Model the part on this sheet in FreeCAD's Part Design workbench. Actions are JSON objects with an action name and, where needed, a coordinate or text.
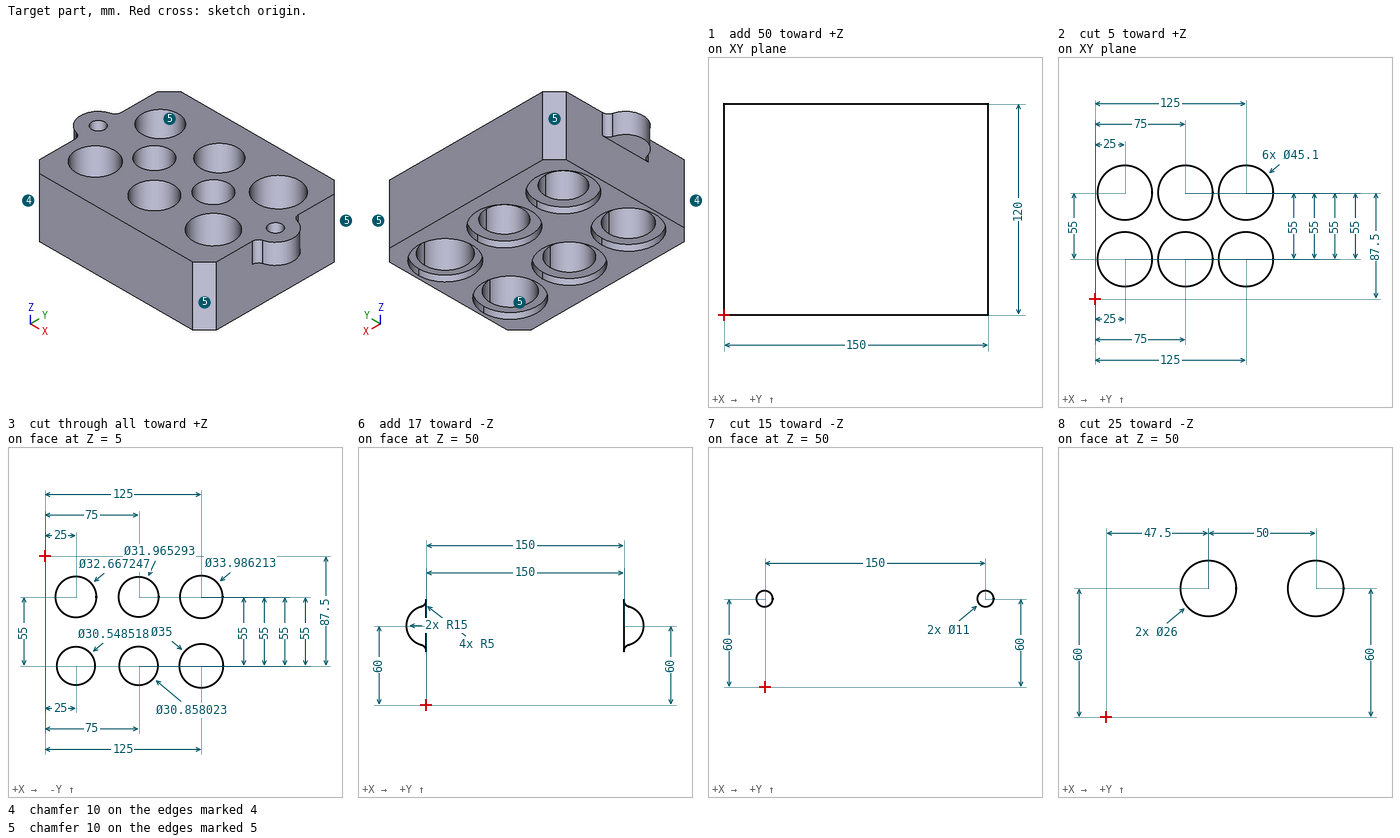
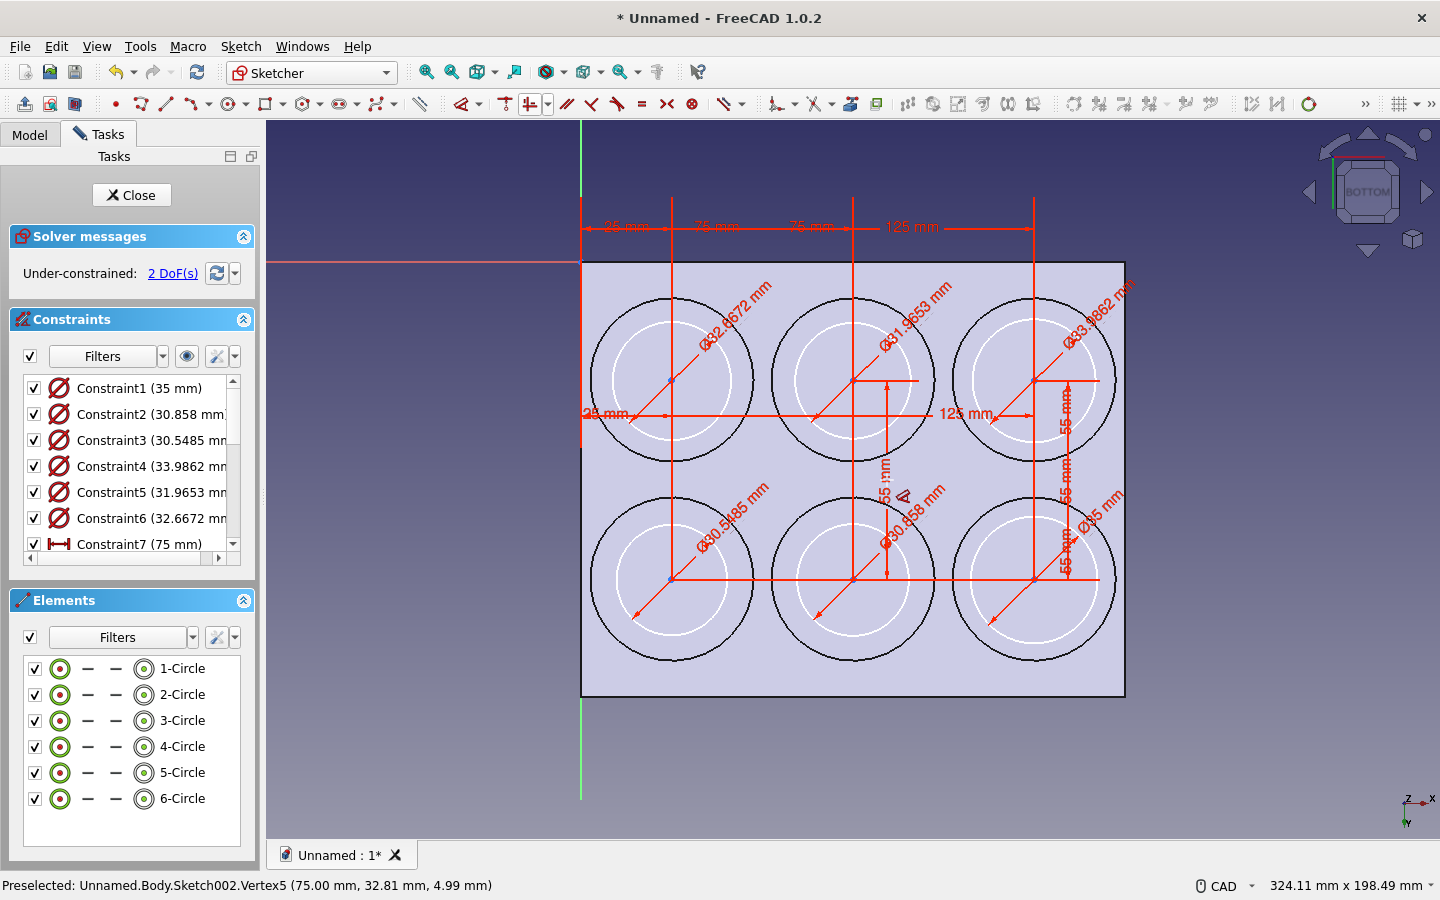
{"action": "left_click", "coordinate": [672, 580]}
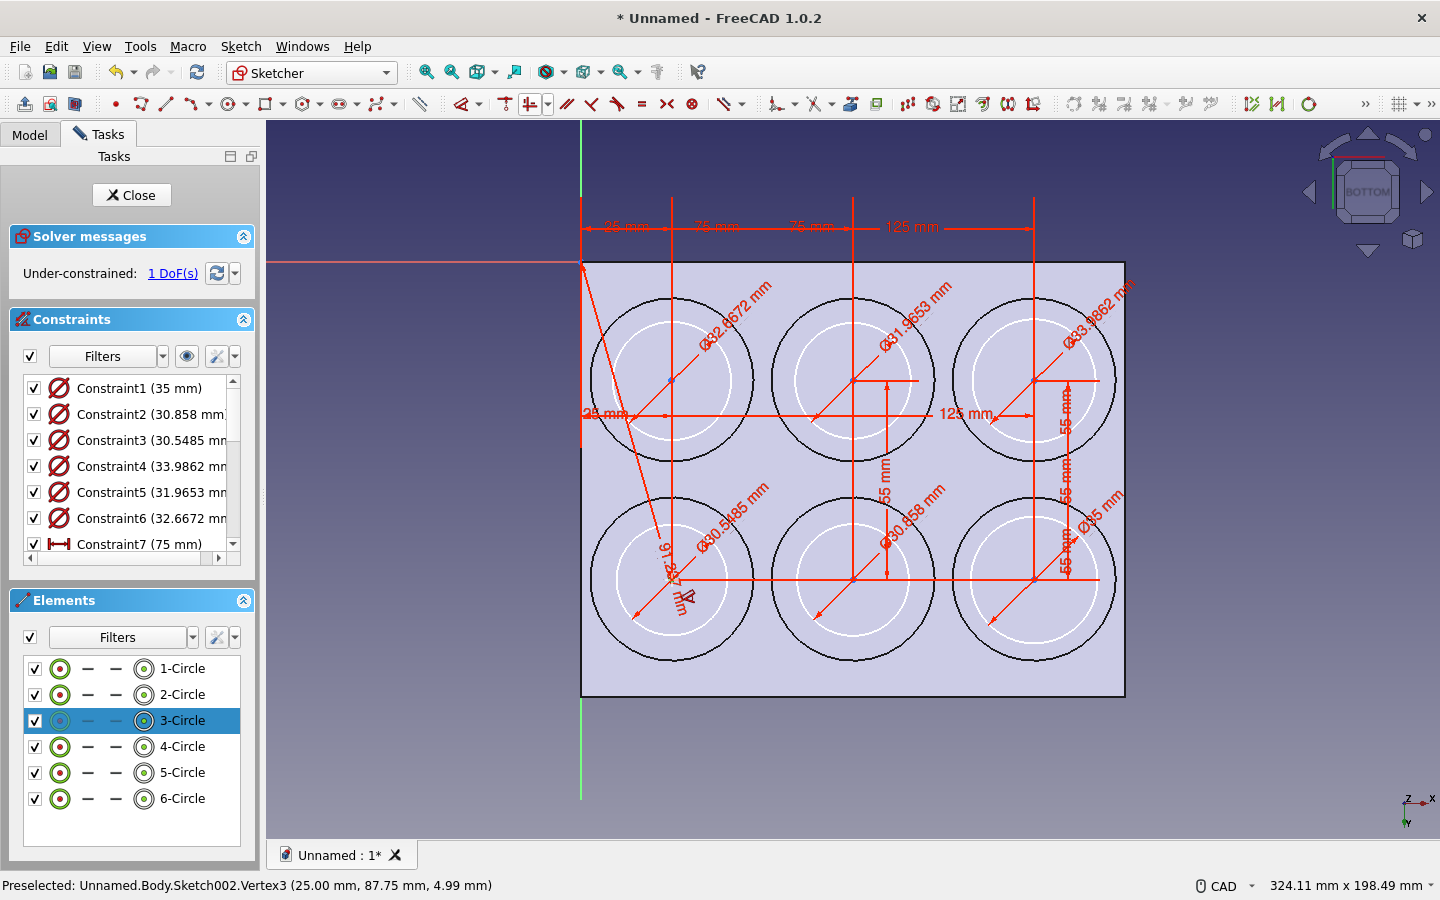
{"action": "left_click", "coordinate": [672, 381]}
{"action": "left_click", "coordinate": [638, 480]}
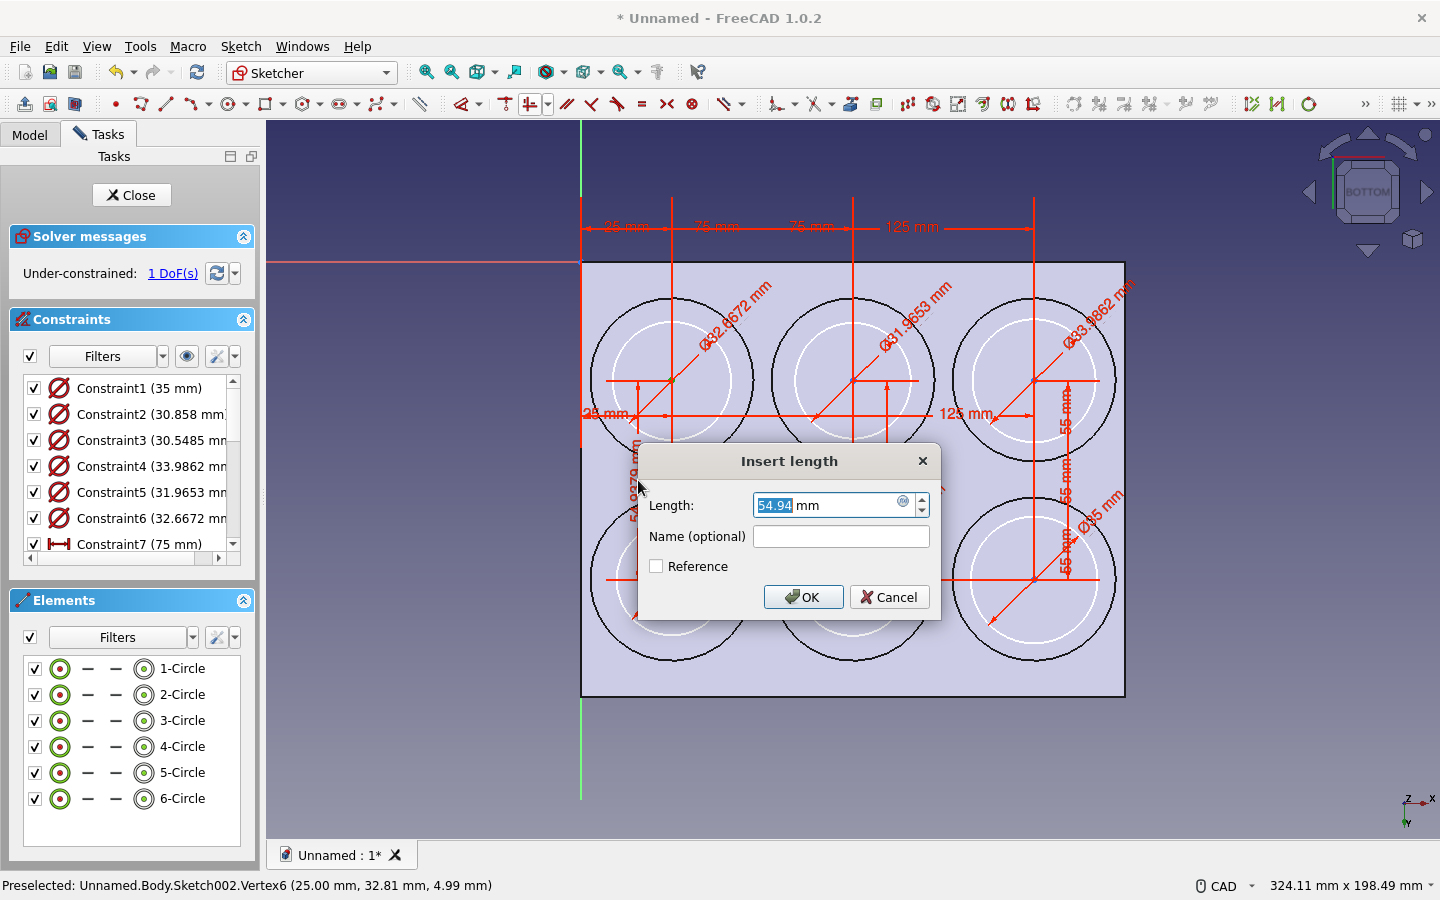
{"action": "type", "text": "55"}
{"action": "key", "text": "Return"}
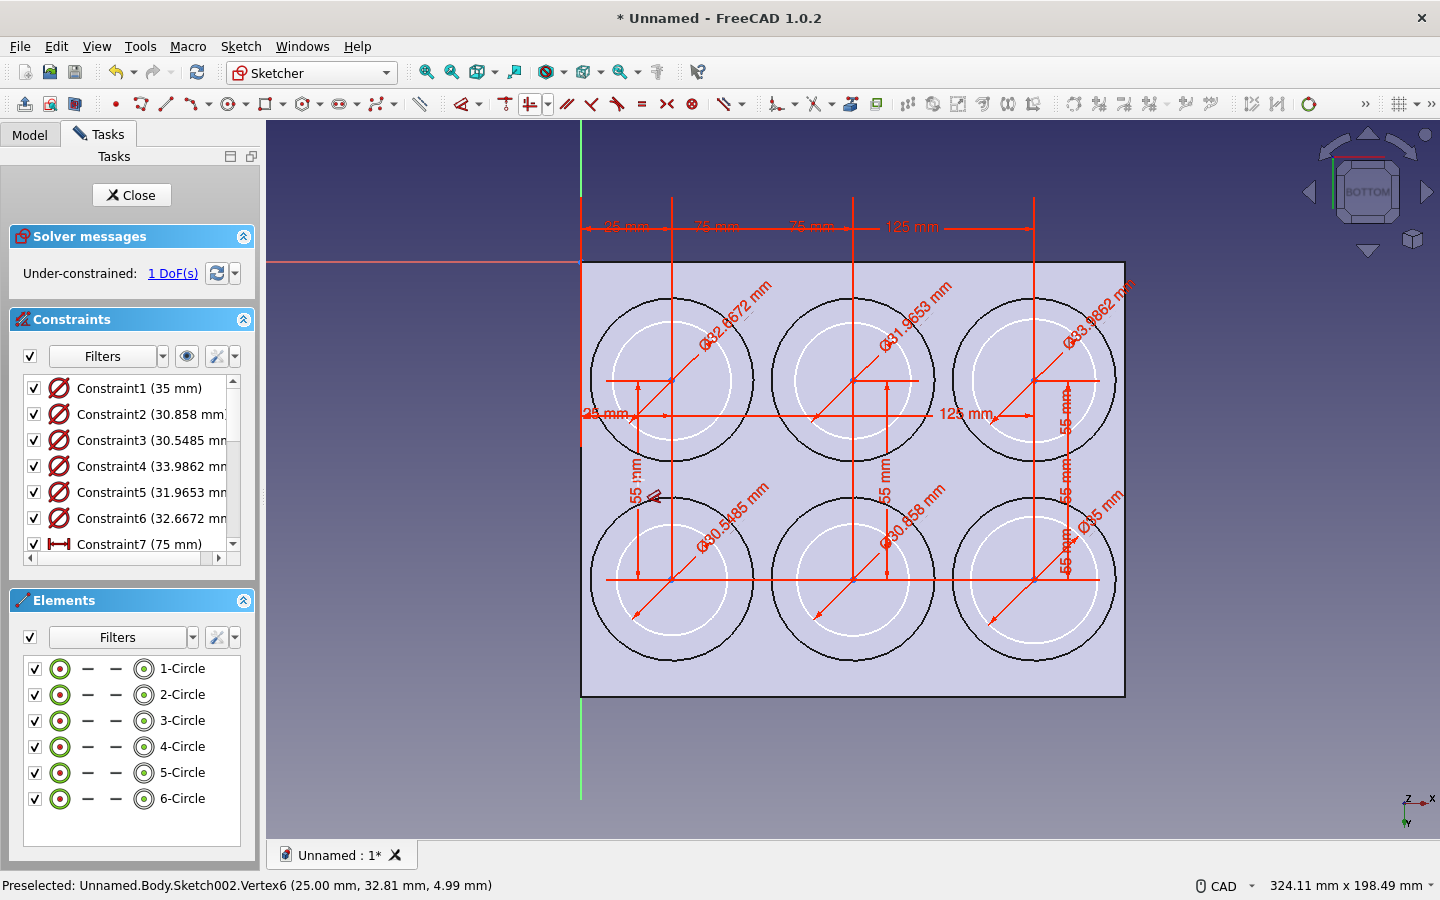
{"action": "left_click", "coordinate": [1034, 580]}
{"action": "left_click", "coordinate": [547, 348]}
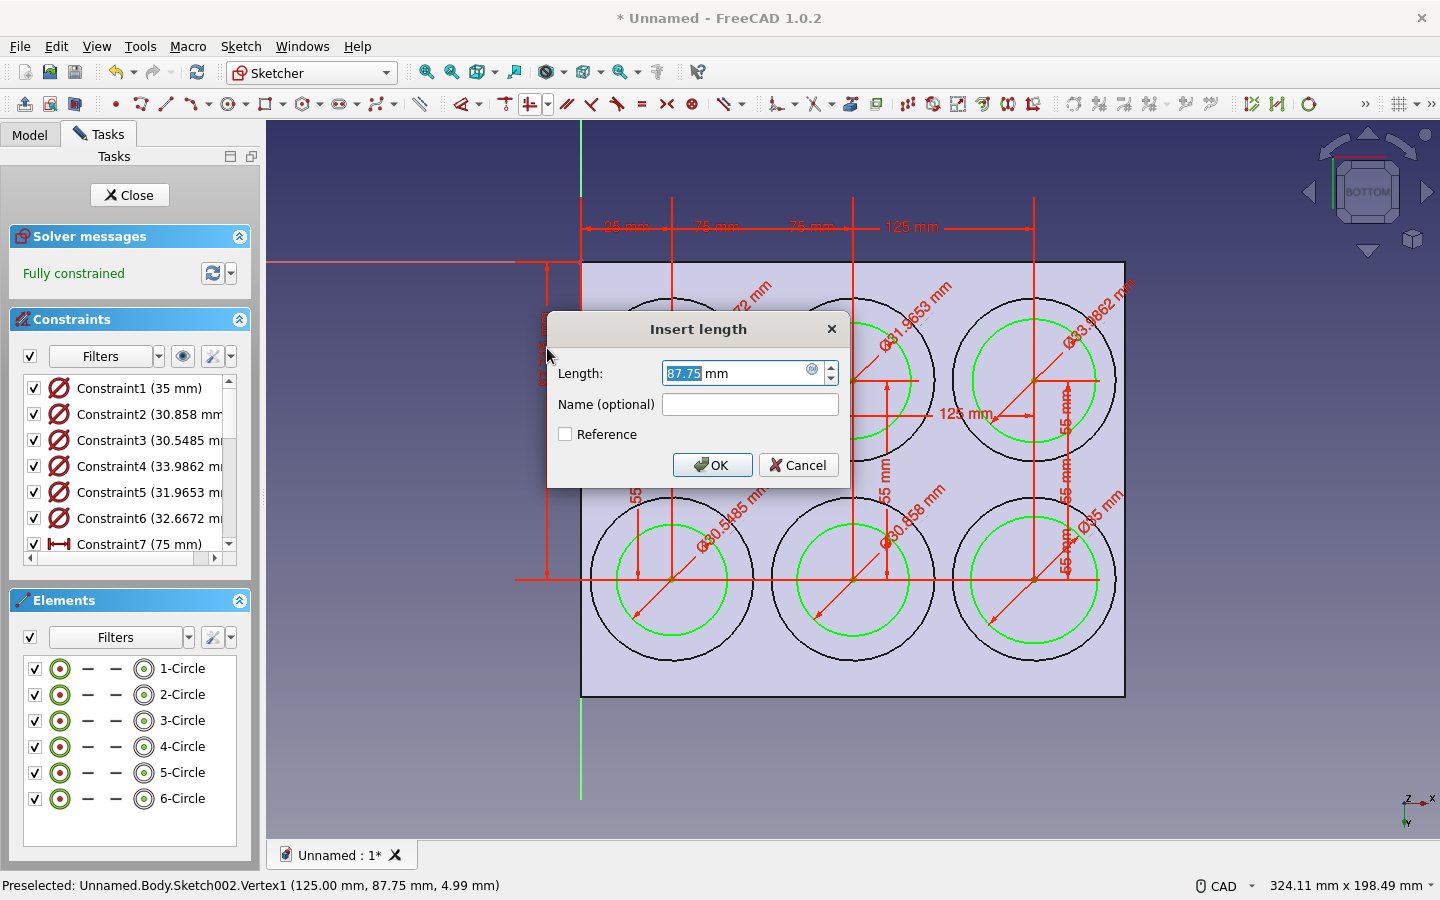
{"action": "type", "text": "87.5"}
{"action": "key", "text": "Return"}
{"action": "key", "text": "Escape"}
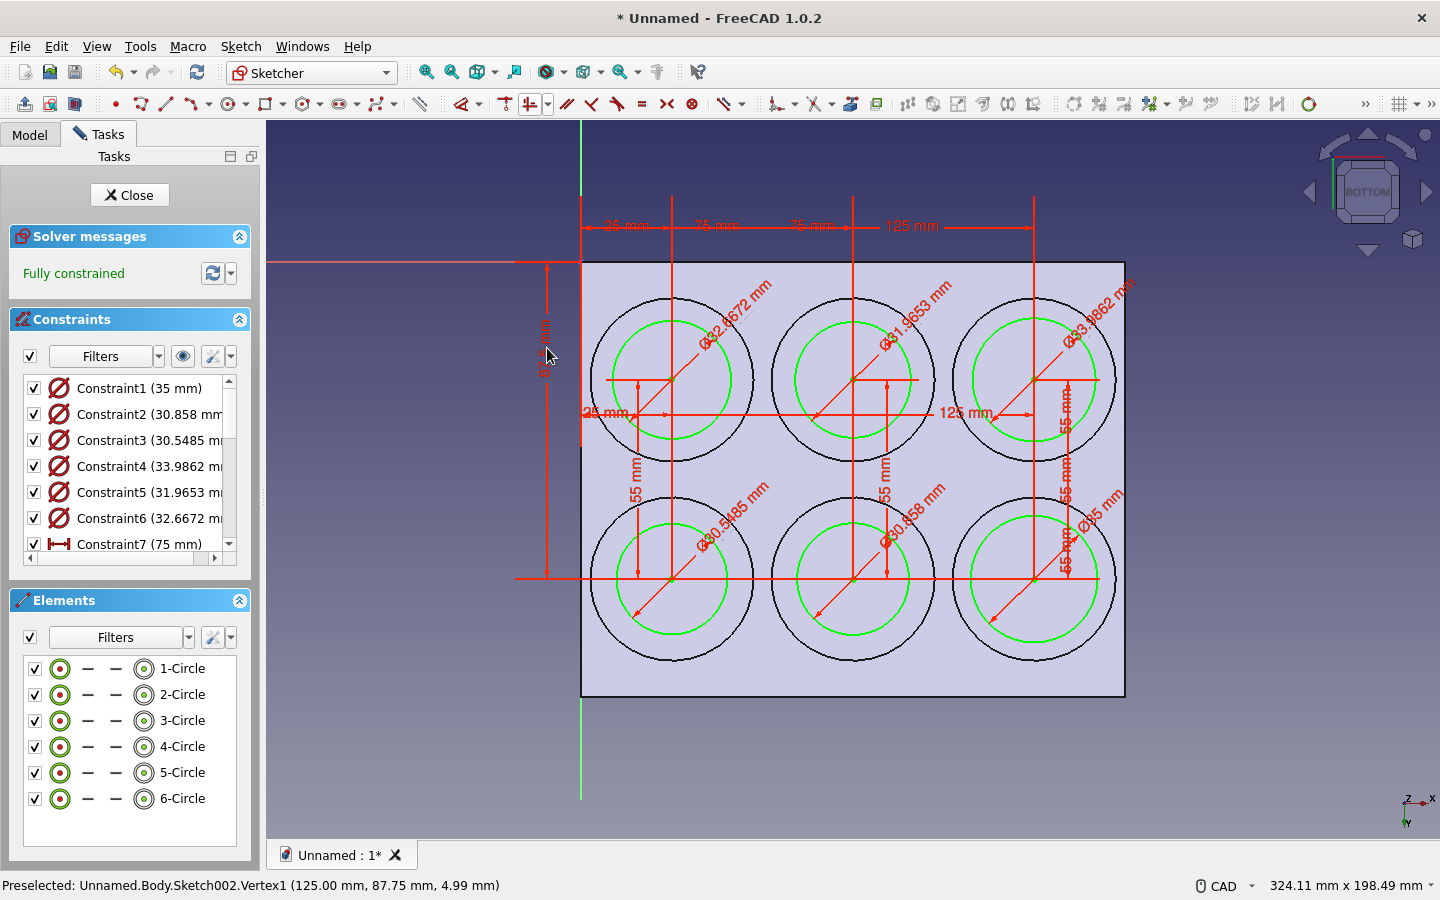
{"action": "left_click", "coordinate": [130, 195]}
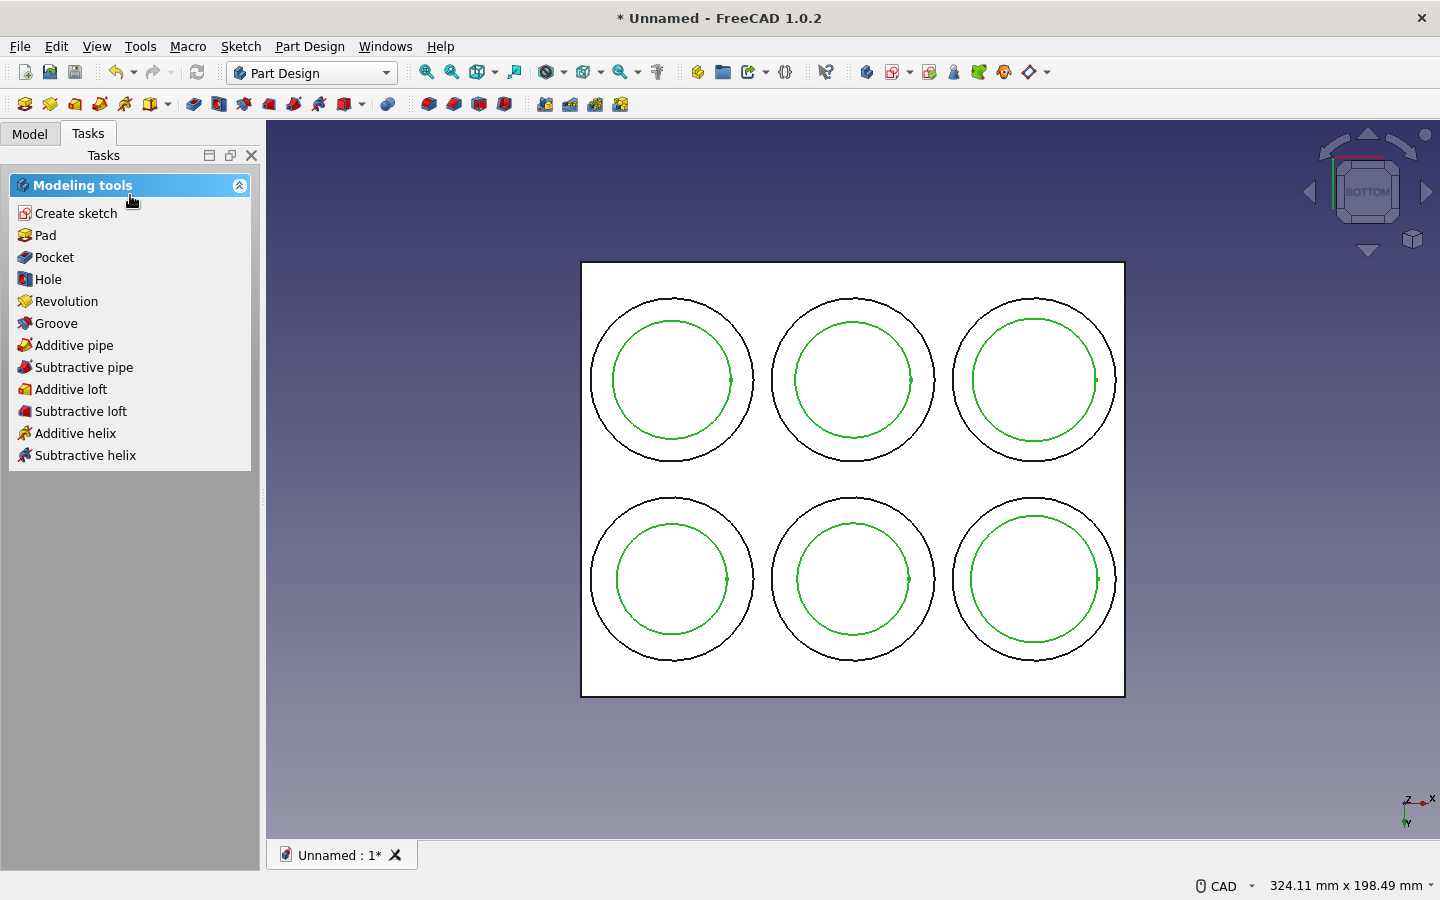
{"action": "left_click", "coordinate": [194, 104]}